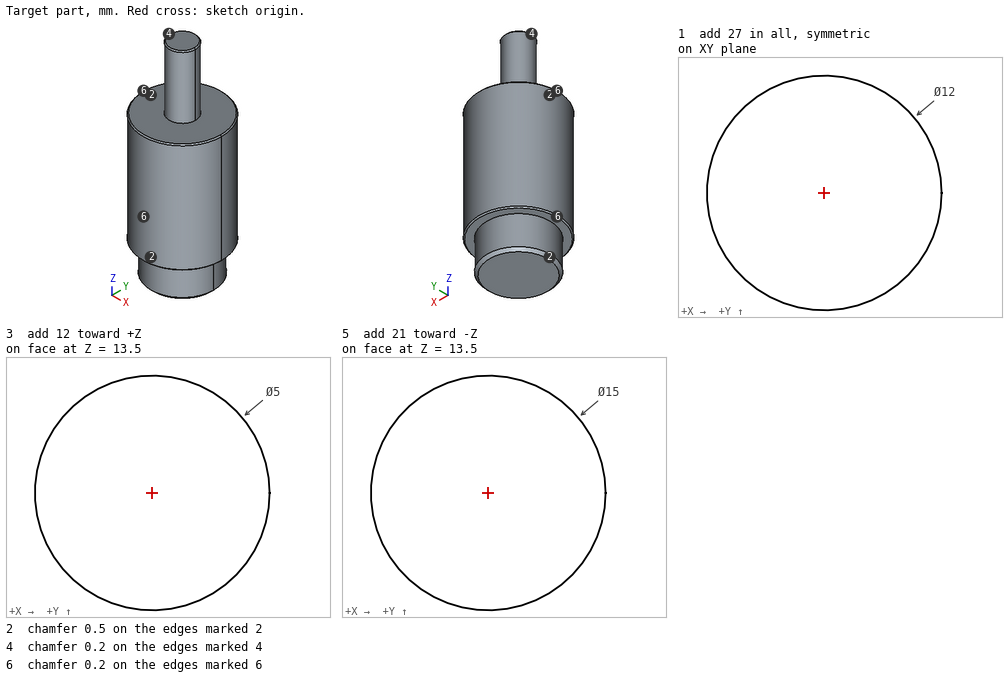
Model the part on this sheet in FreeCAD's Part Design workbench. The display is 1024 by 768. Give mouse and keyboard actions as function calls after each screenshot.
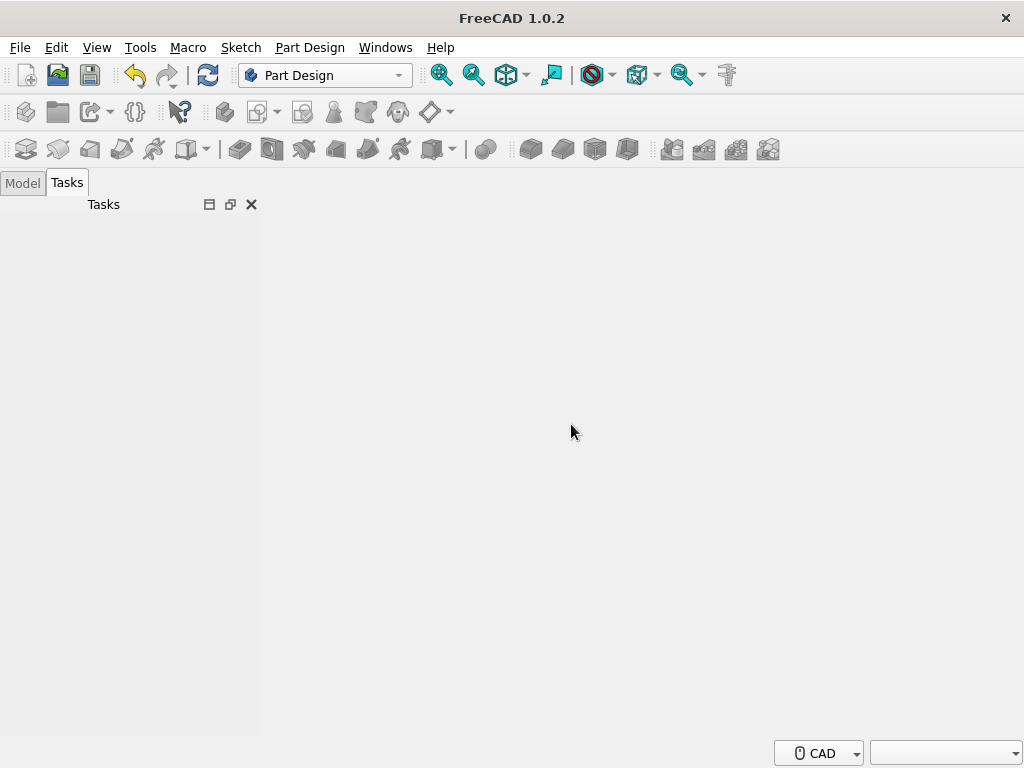
click(26, 76)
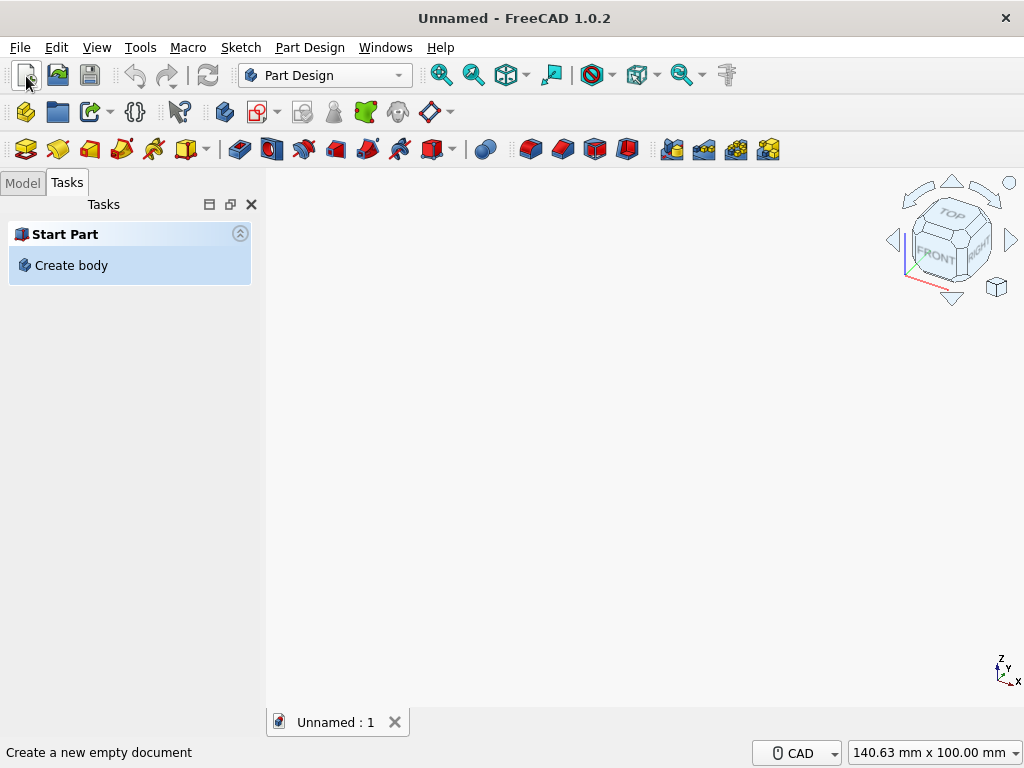
click(258, 112)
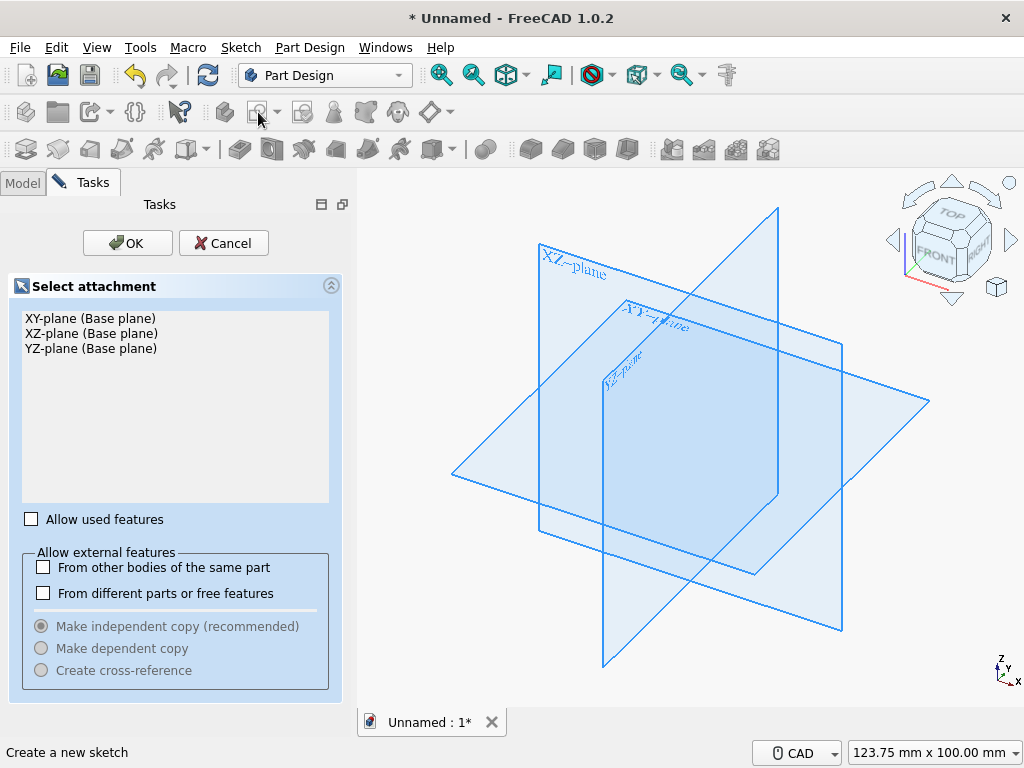
click(82, 318)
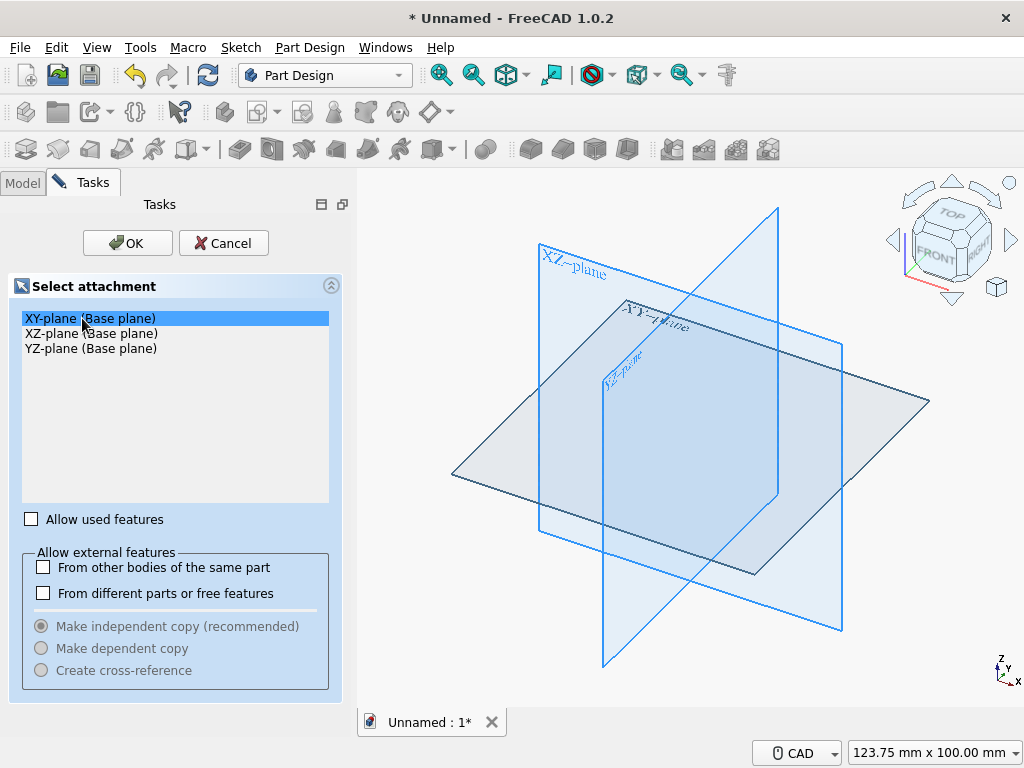
click(128, 243)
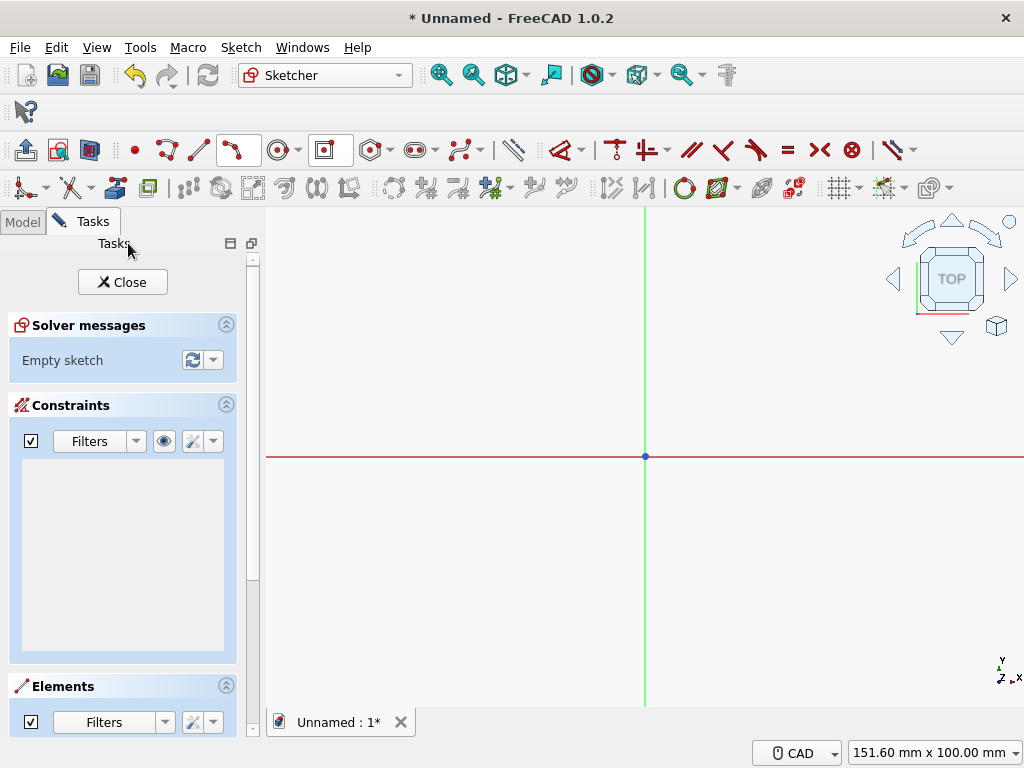
scroll(662, 457, up, 8)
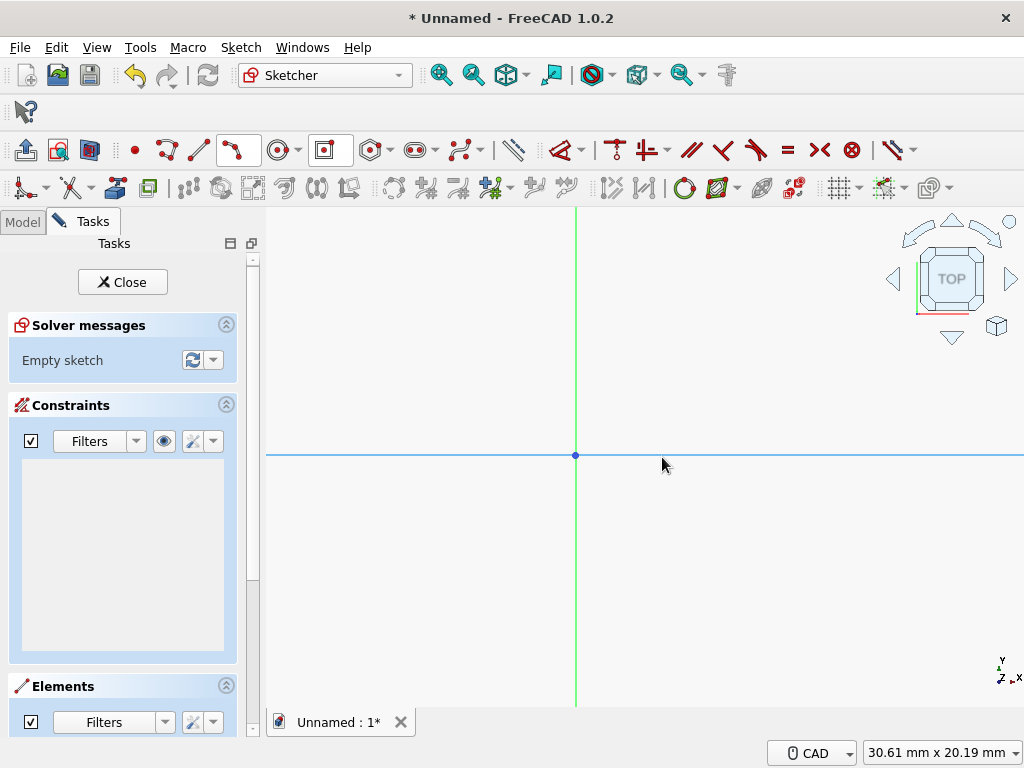
click(278, 150)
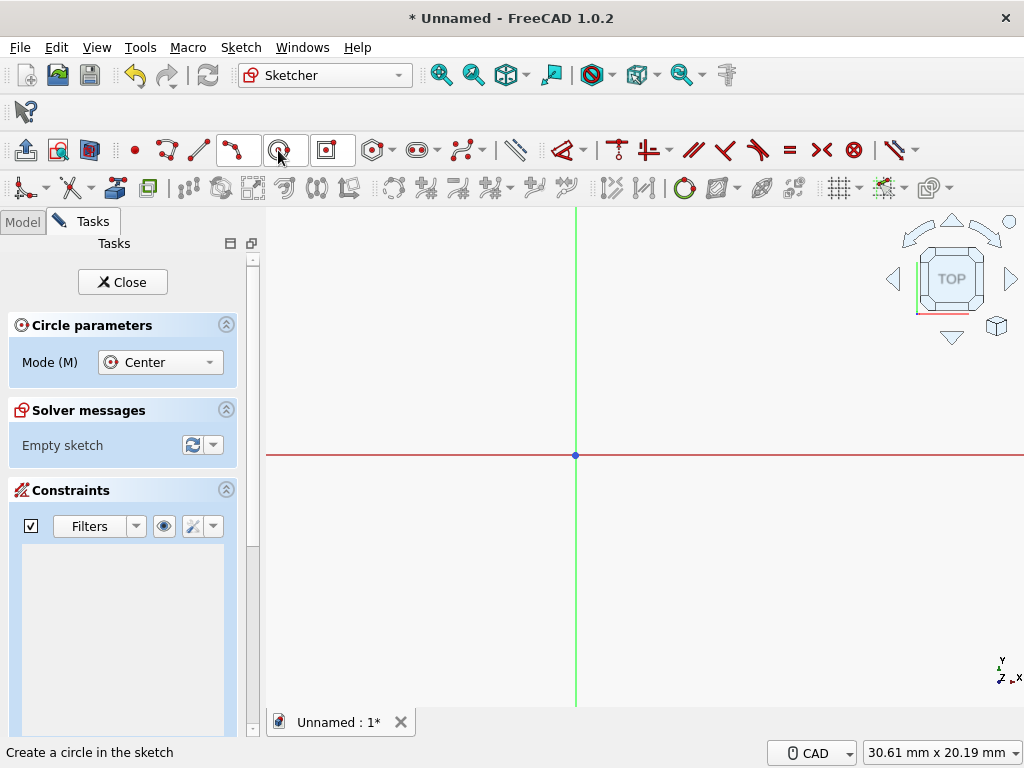
click(576, 455)
move(681, 350)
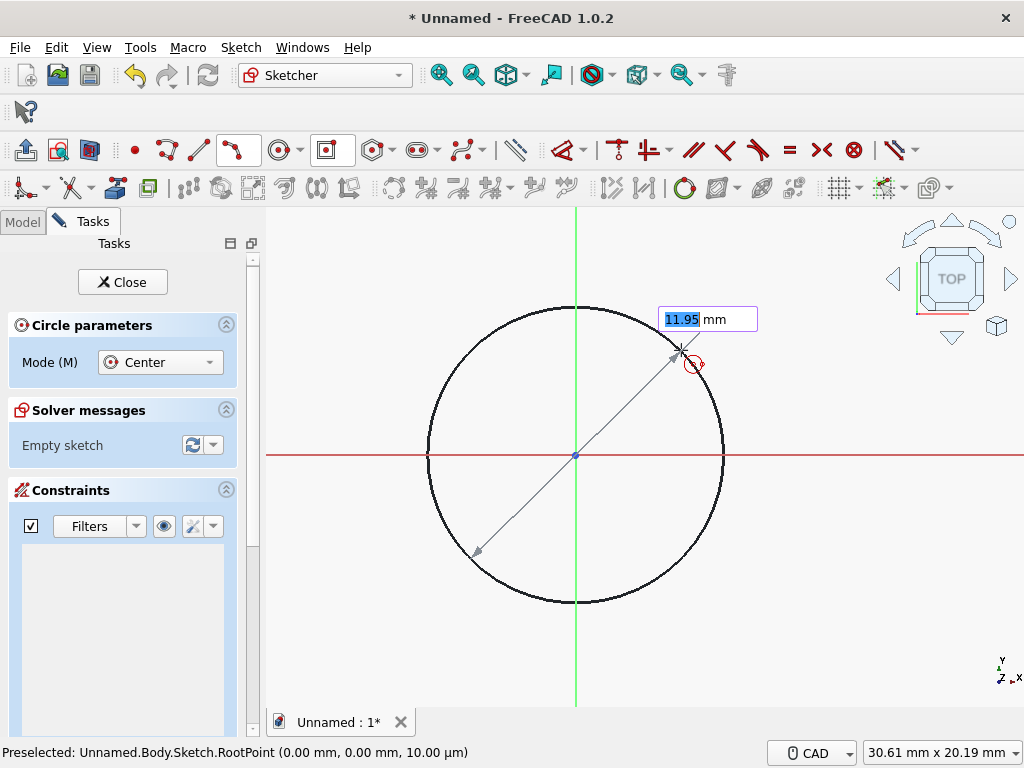
text(12)
key(Return)
key(Escape)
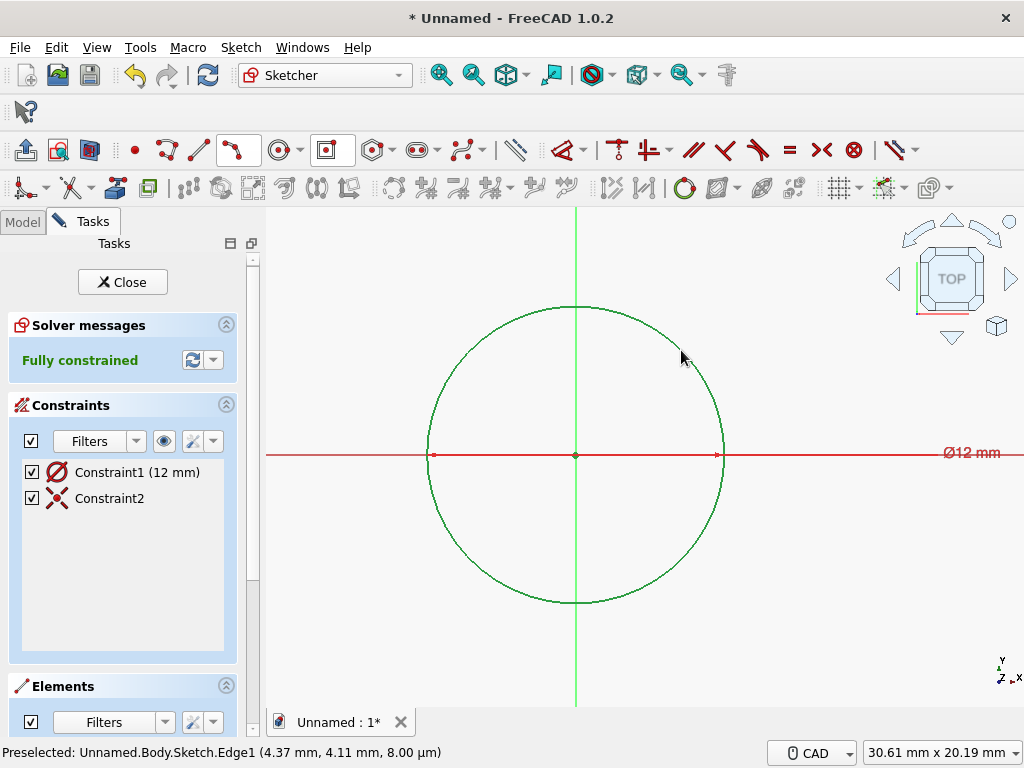
click(123, 282)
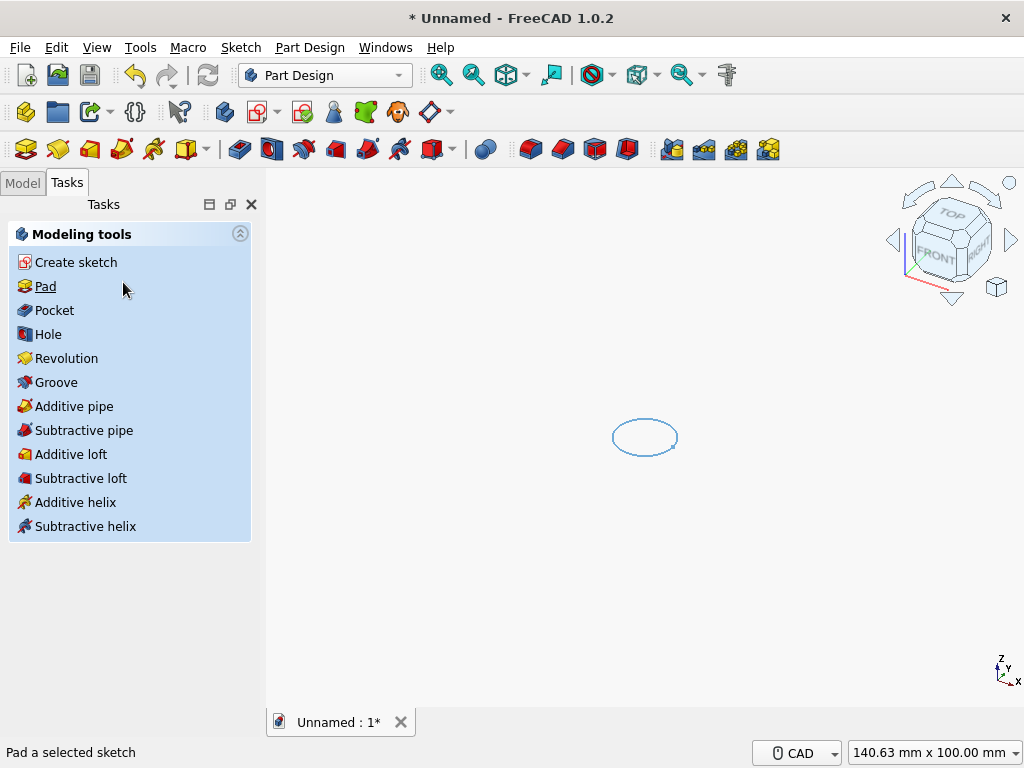
click(26, 150)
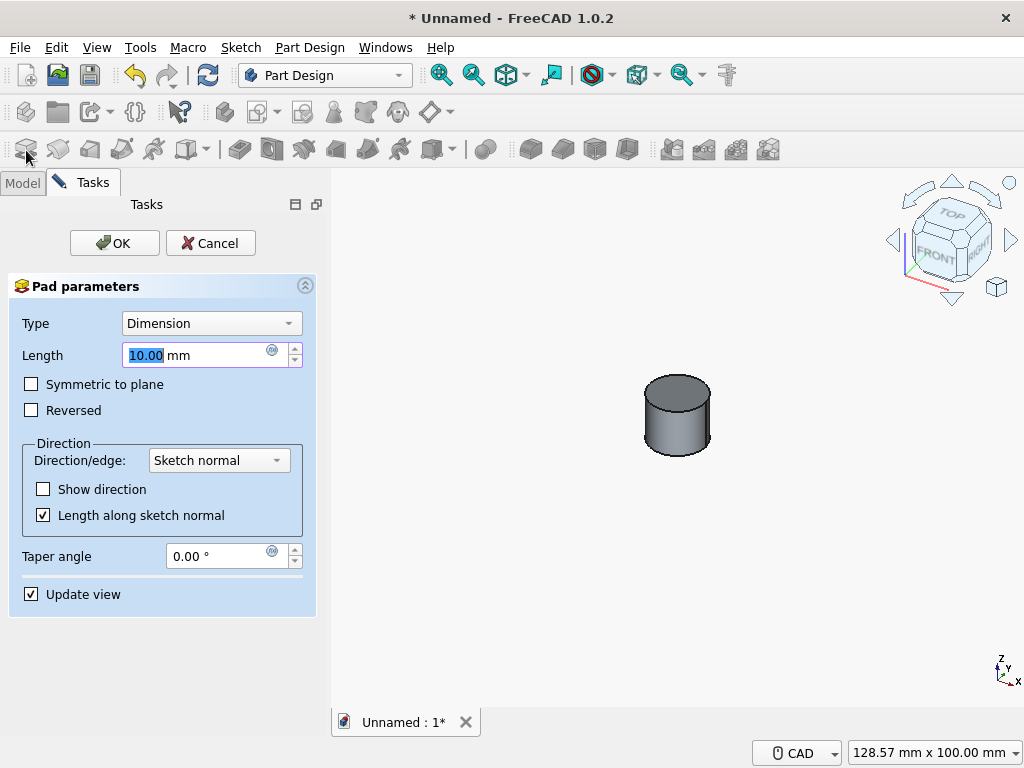
text(27)
key(Tab)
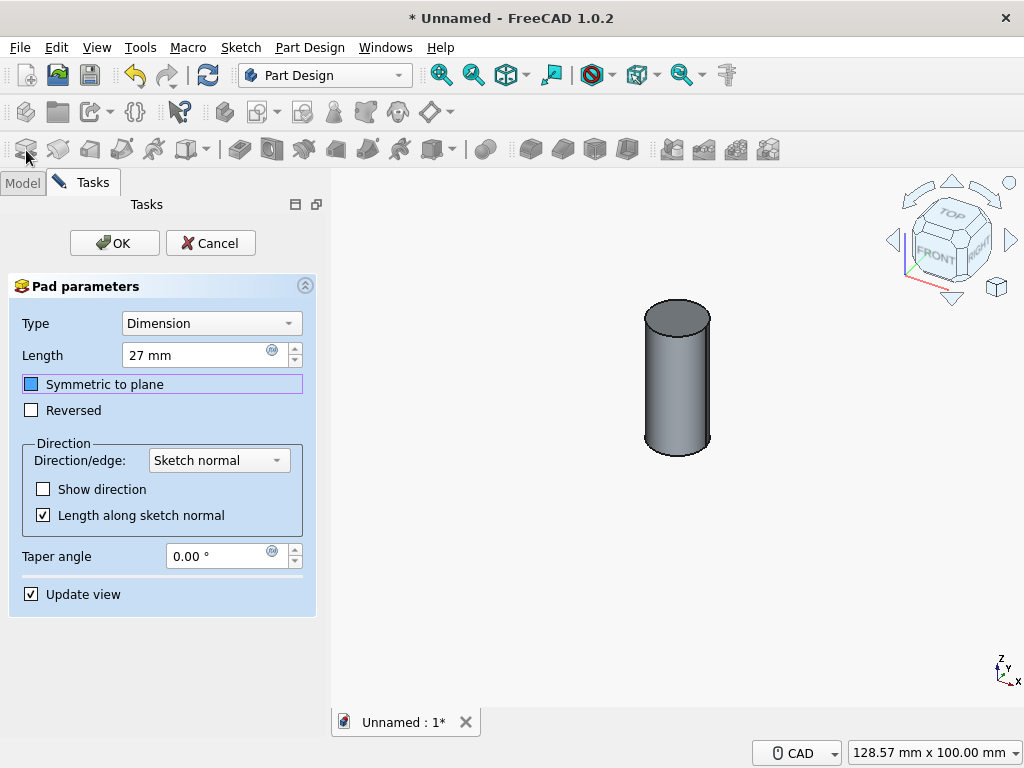
click(30, 384)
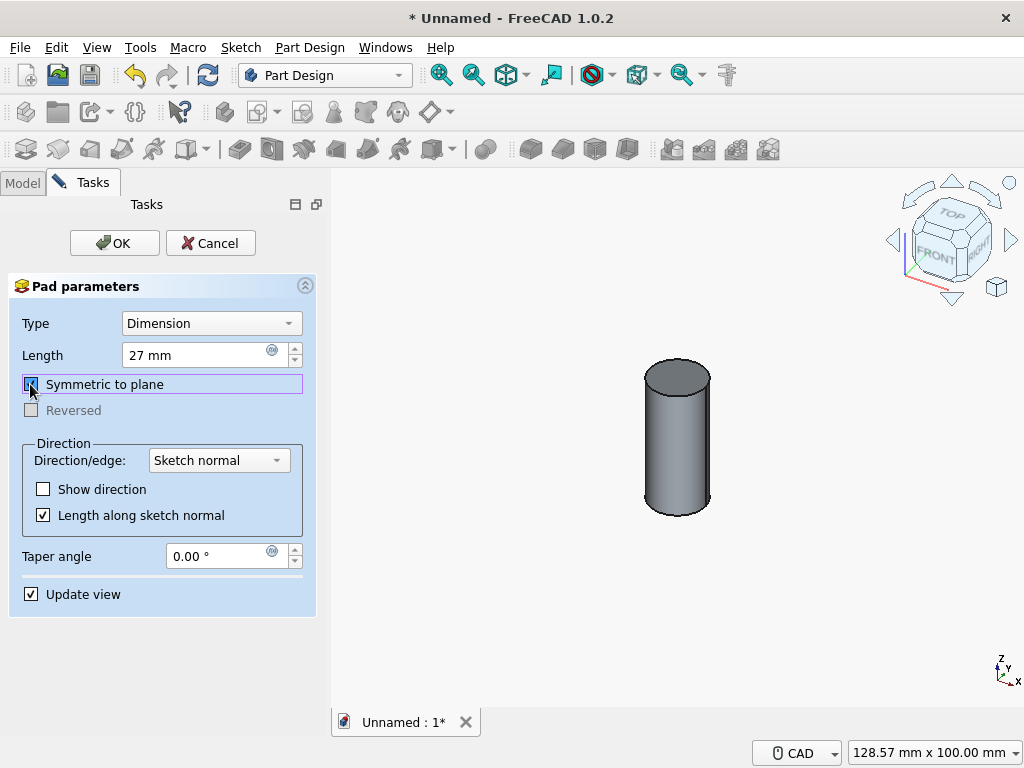
click(115, 243)